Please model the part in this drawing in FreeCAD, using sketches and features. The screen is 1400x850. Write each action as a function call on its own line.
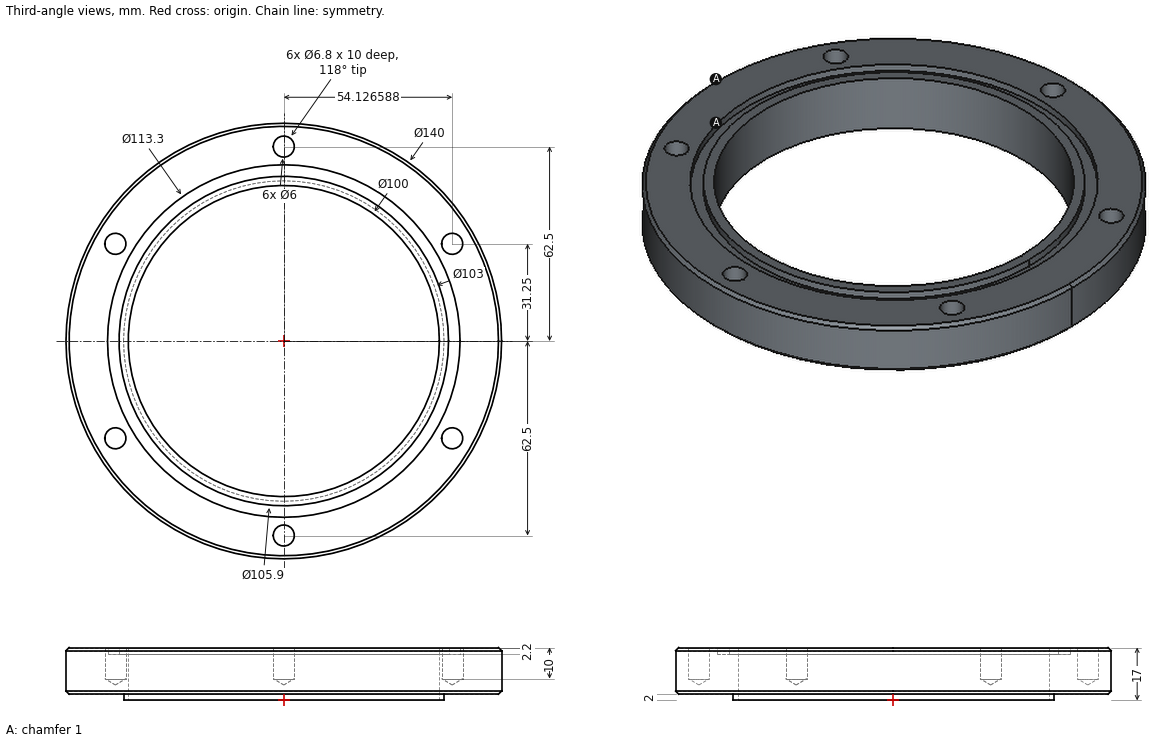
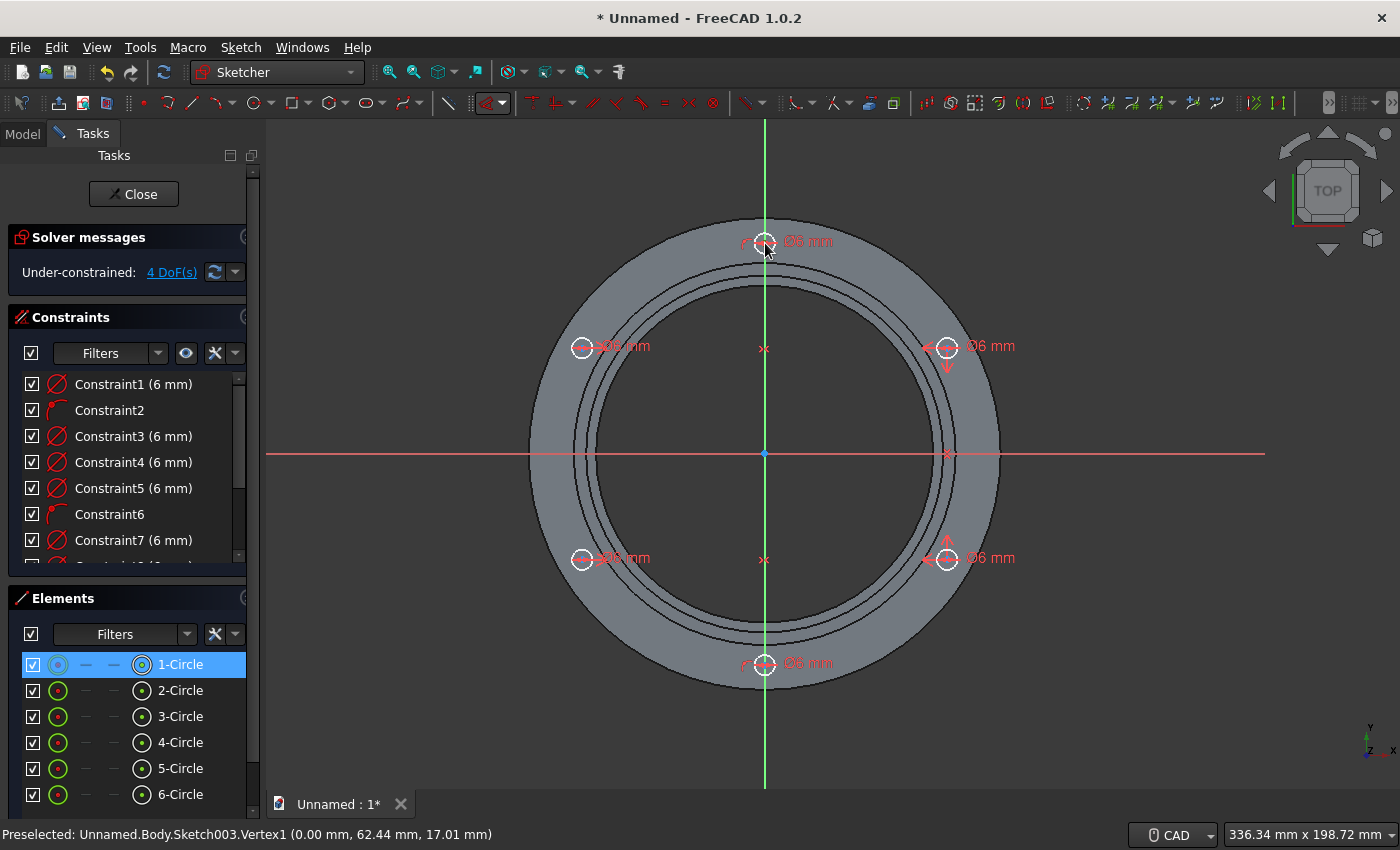
key(i)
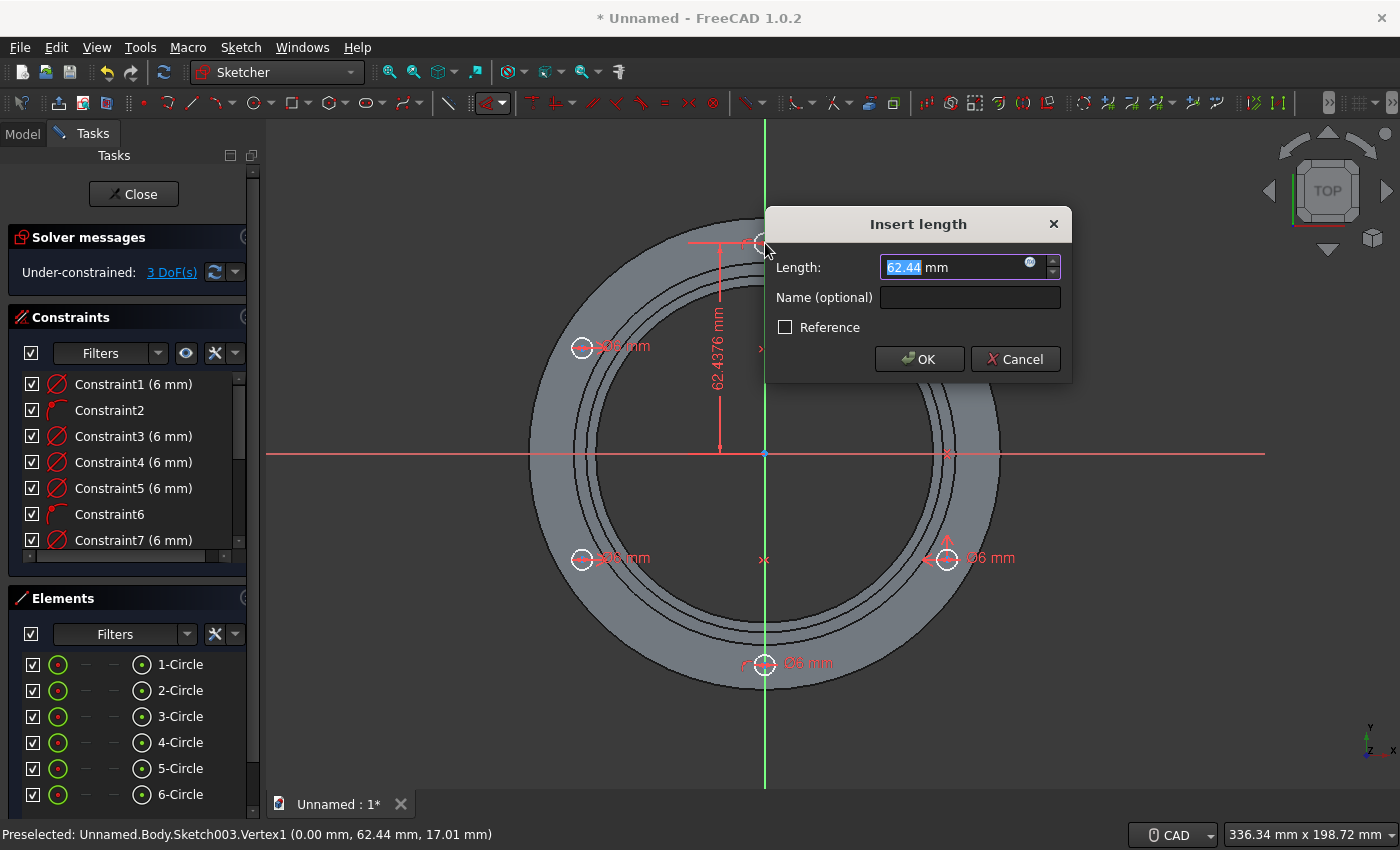
text(62.5)
key(Return)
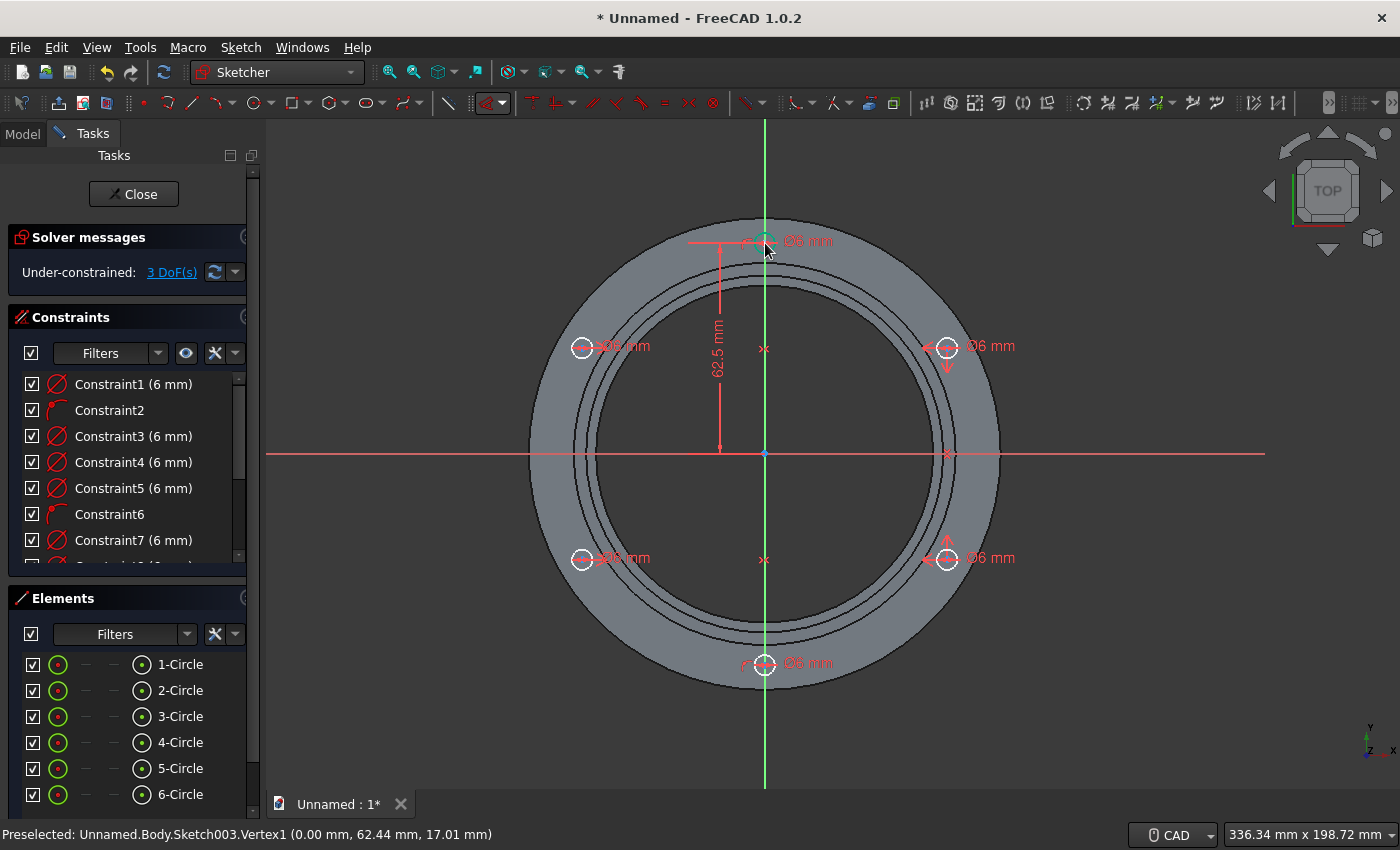
click(765, 665)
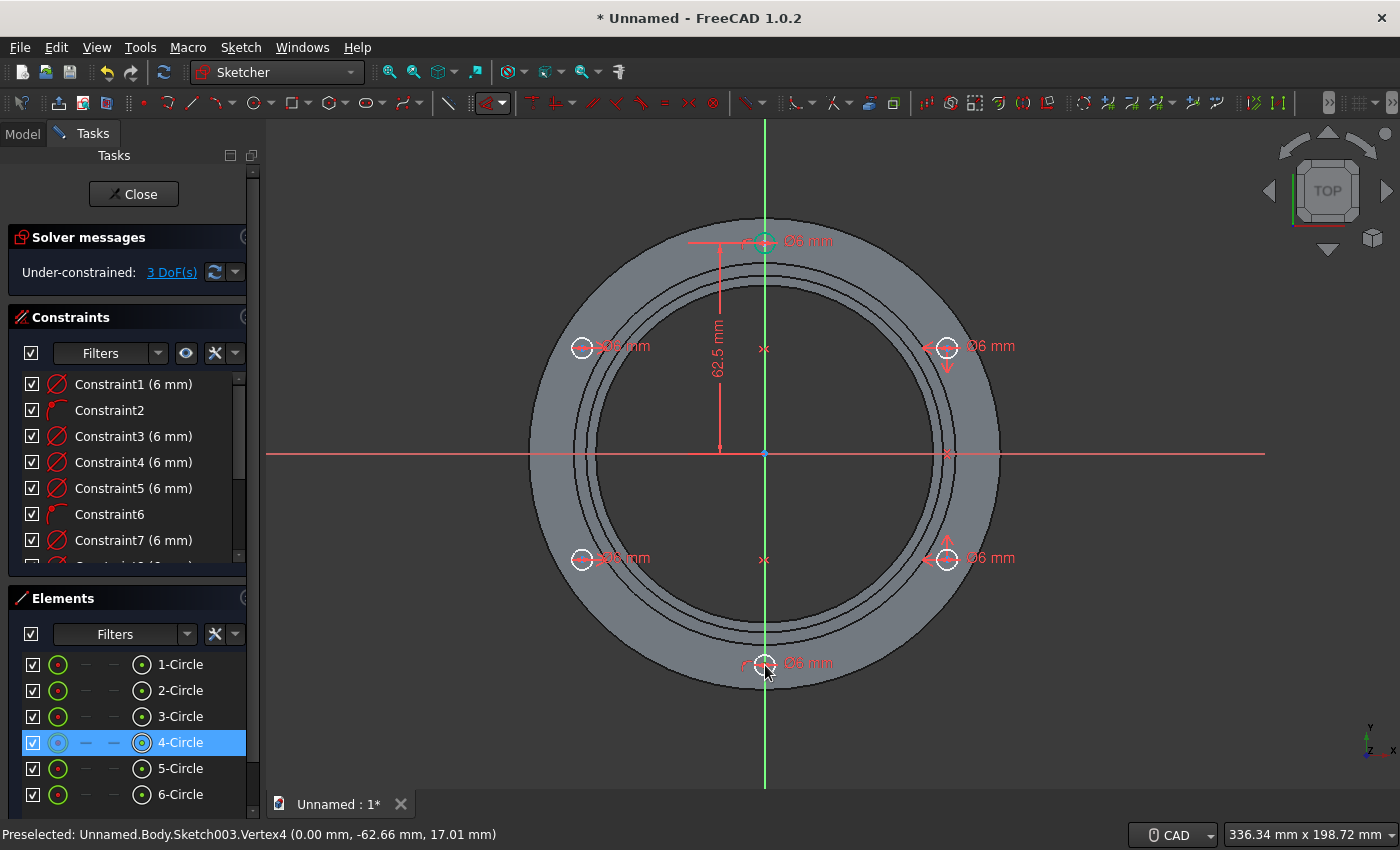
click(504, 104)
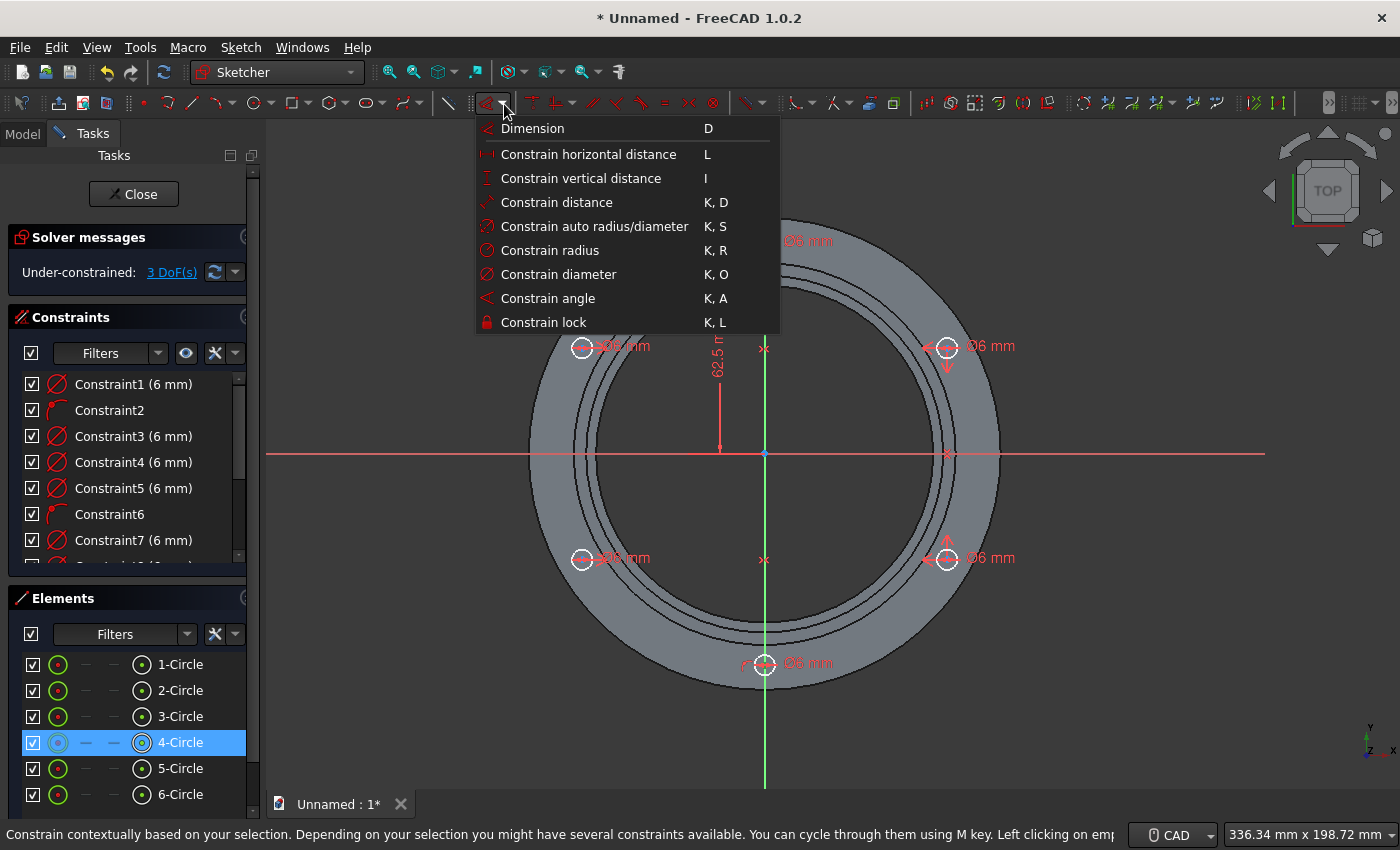
click(628, 178)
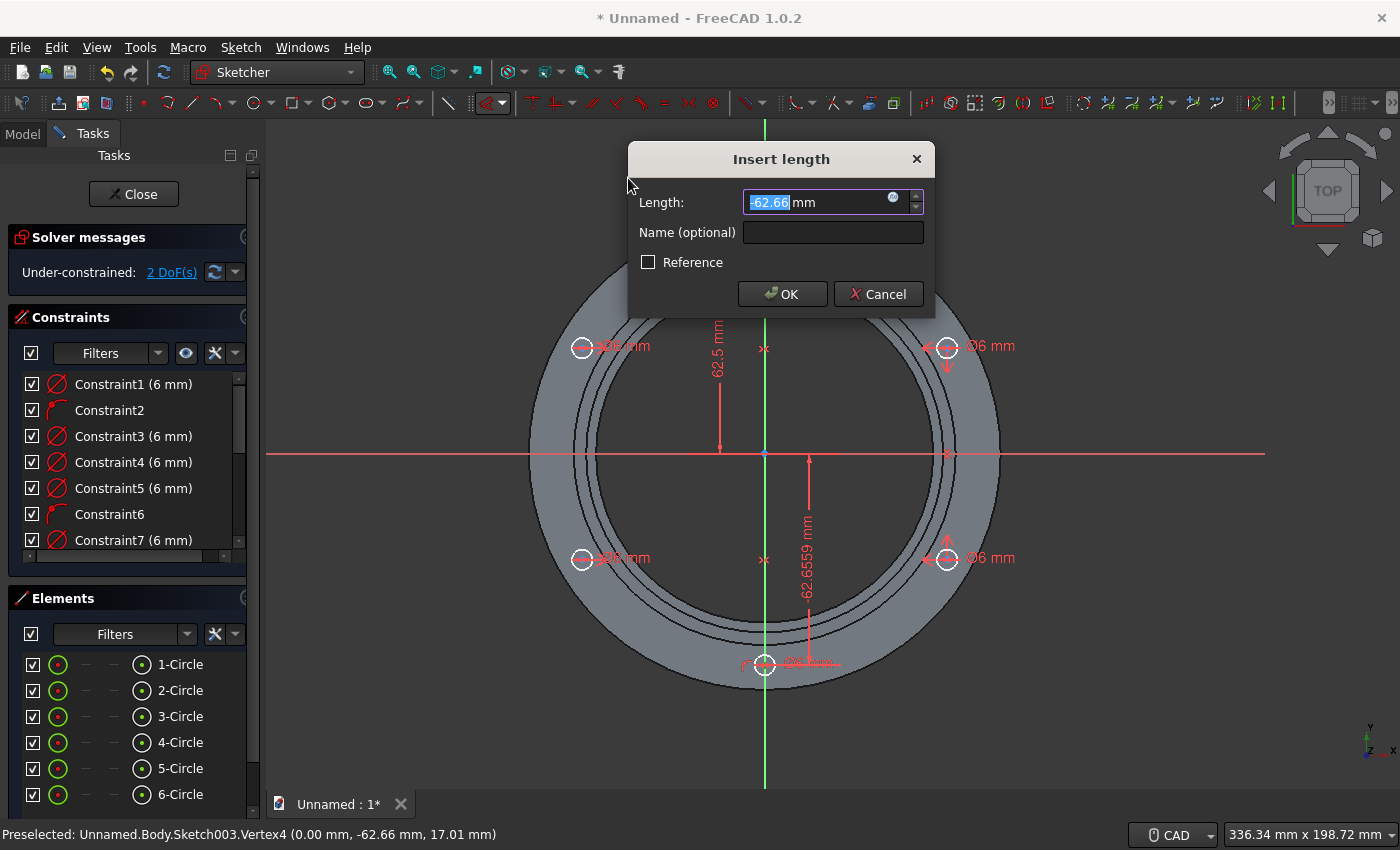
text(-62.5)
key(Return)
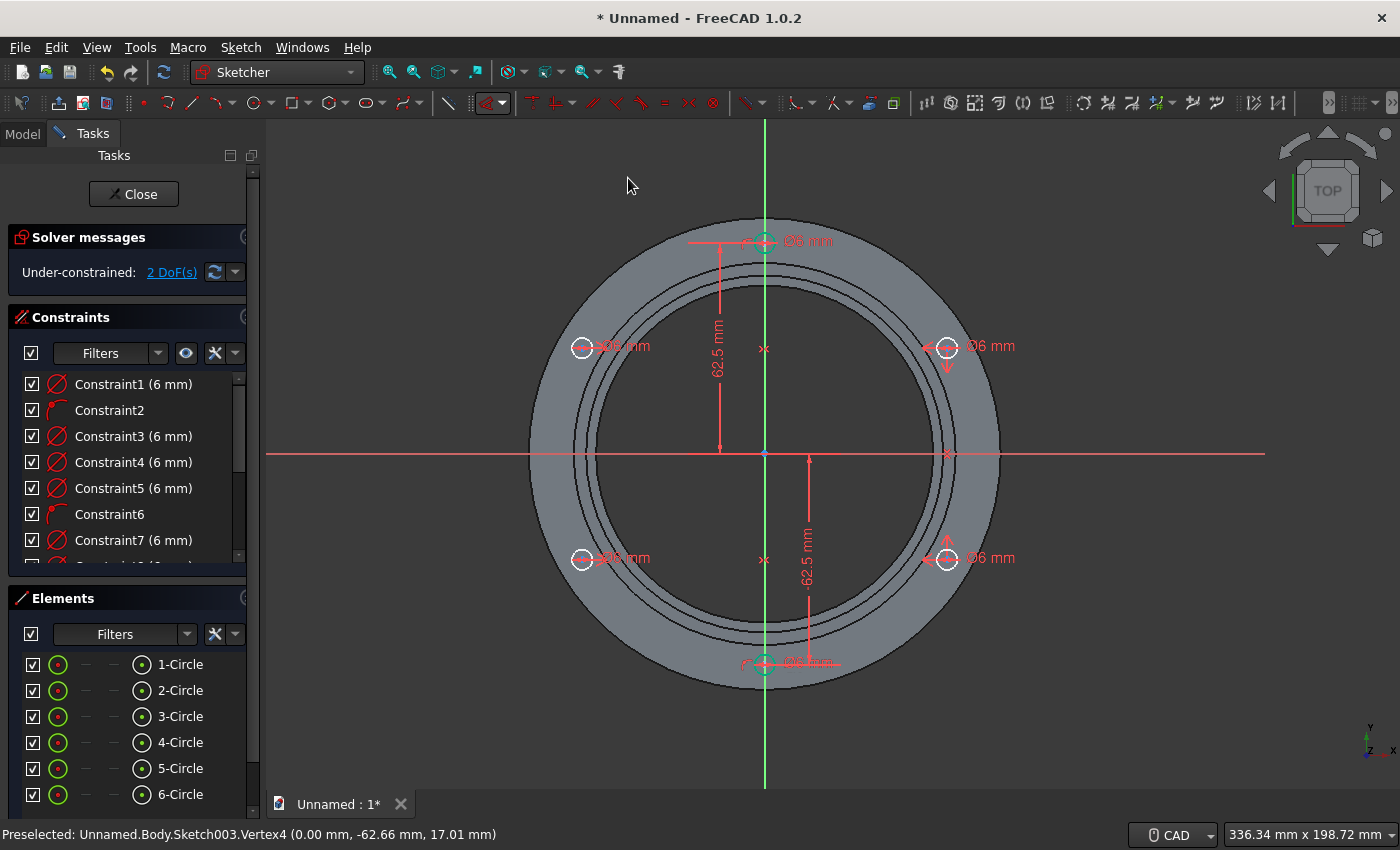
click(947, 348)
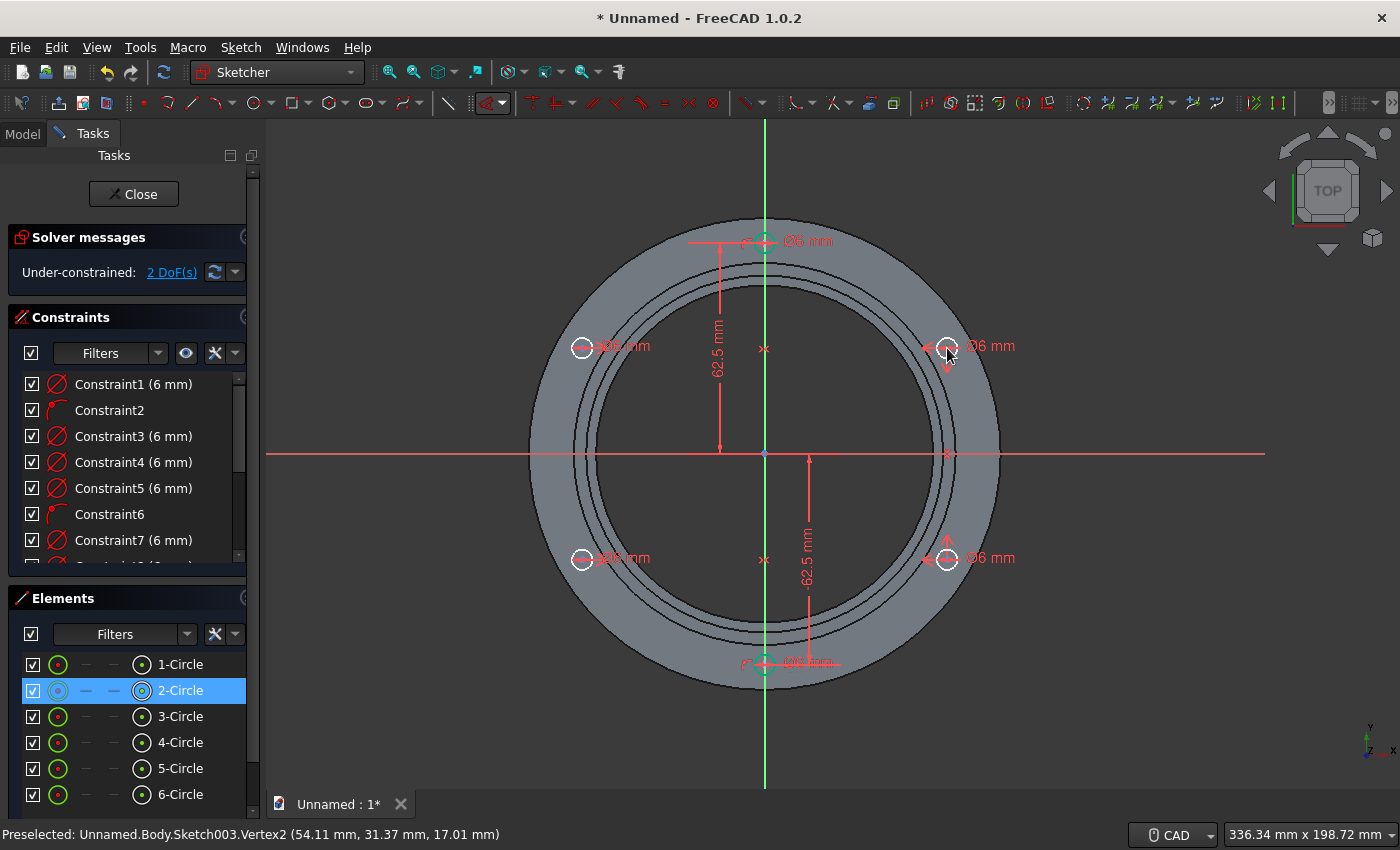
key(i)